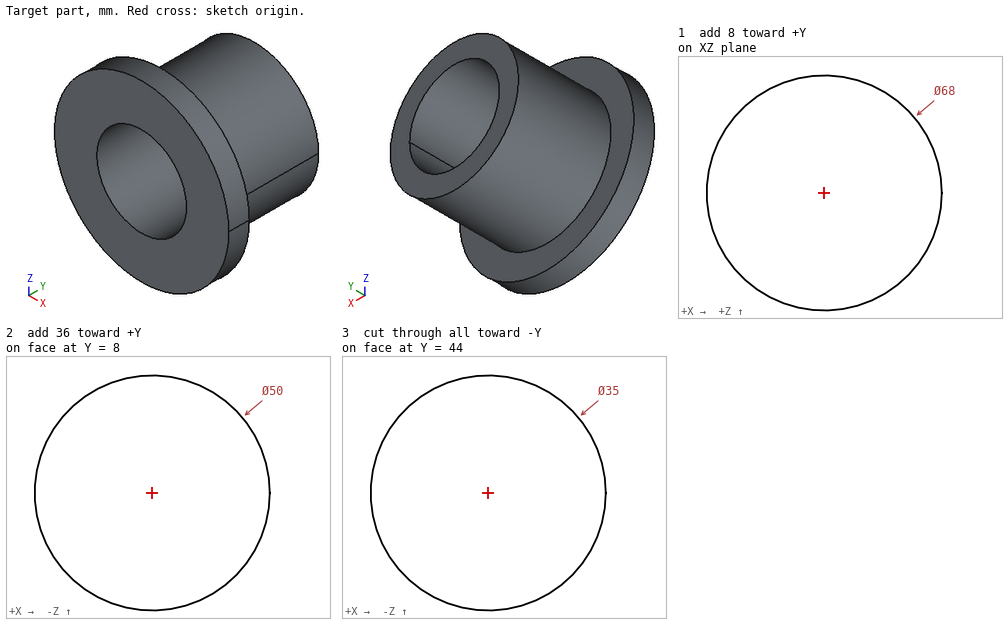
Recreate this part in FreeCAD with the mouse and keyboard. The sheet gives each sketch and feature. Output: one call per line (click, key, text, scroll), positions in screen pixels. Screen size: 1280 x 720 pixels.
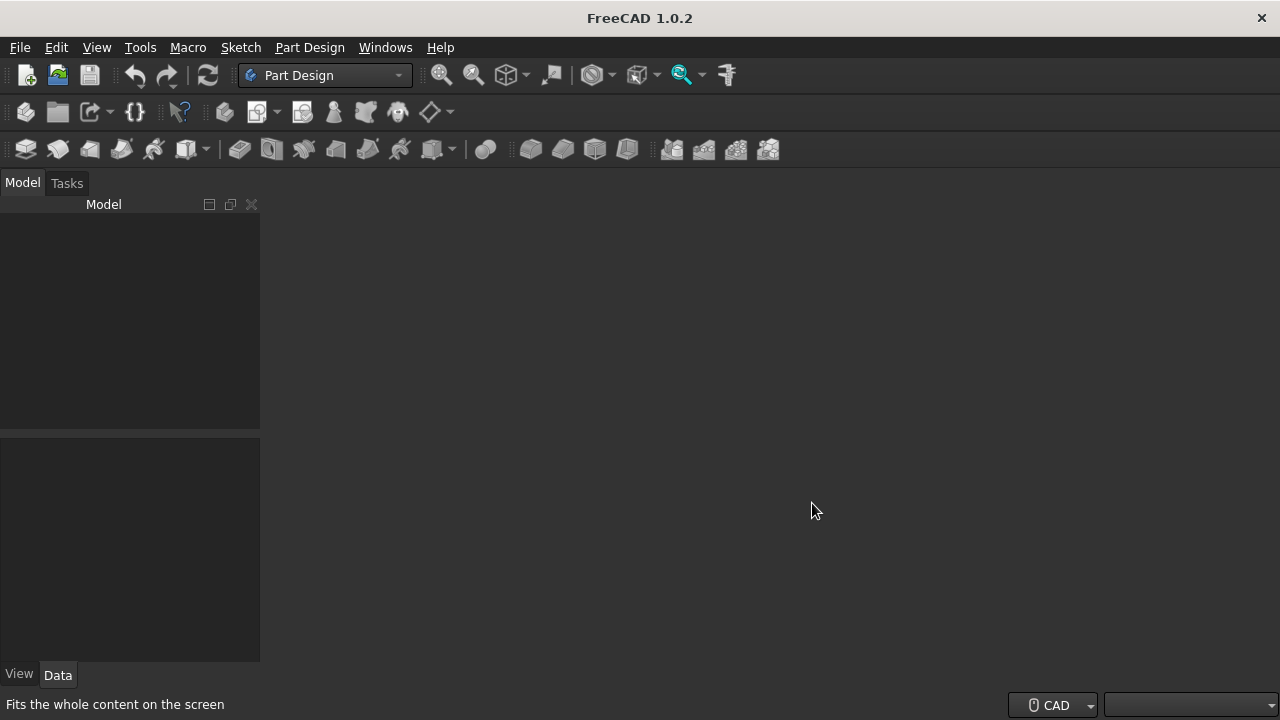
key(ctrl+n)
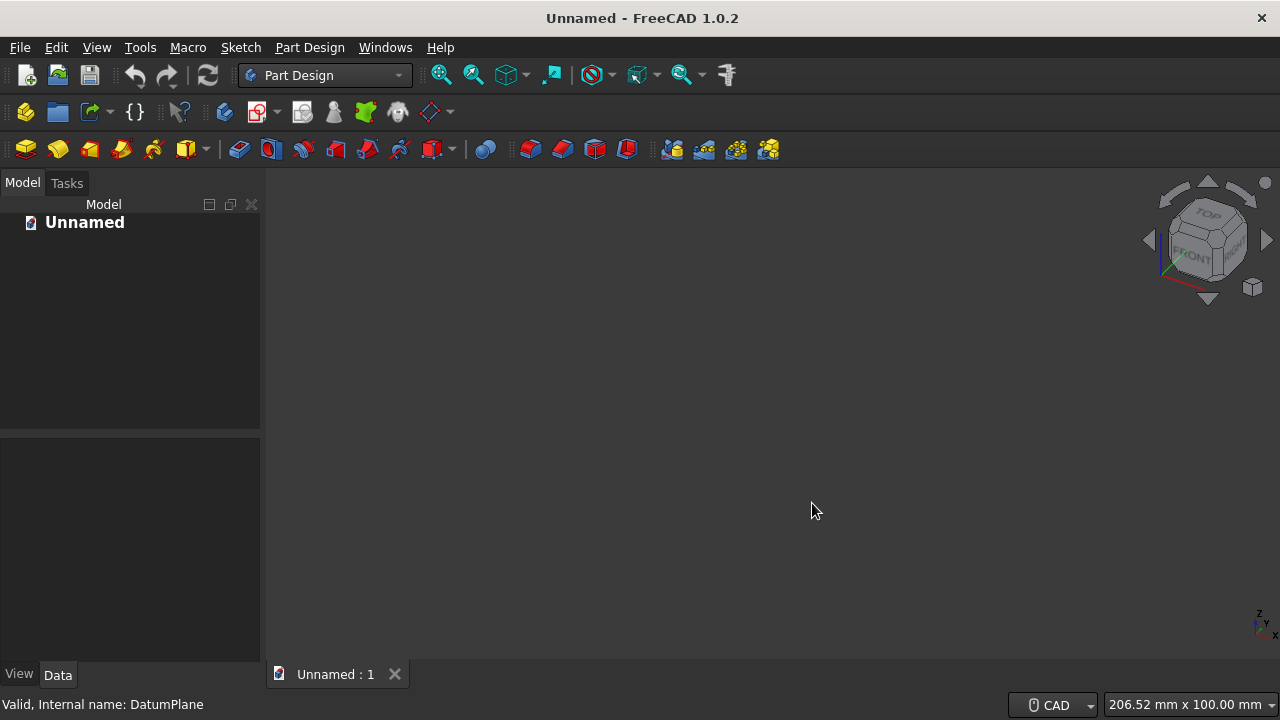
click(258, 112)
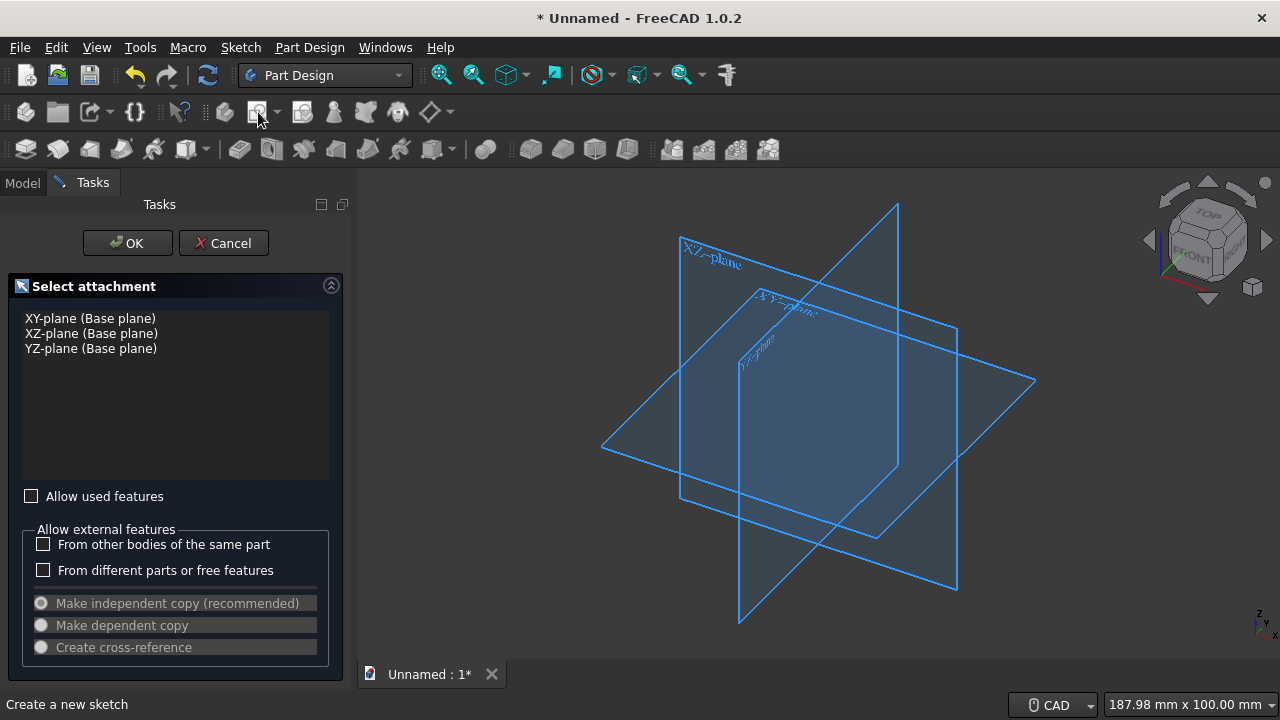
click(82, 334)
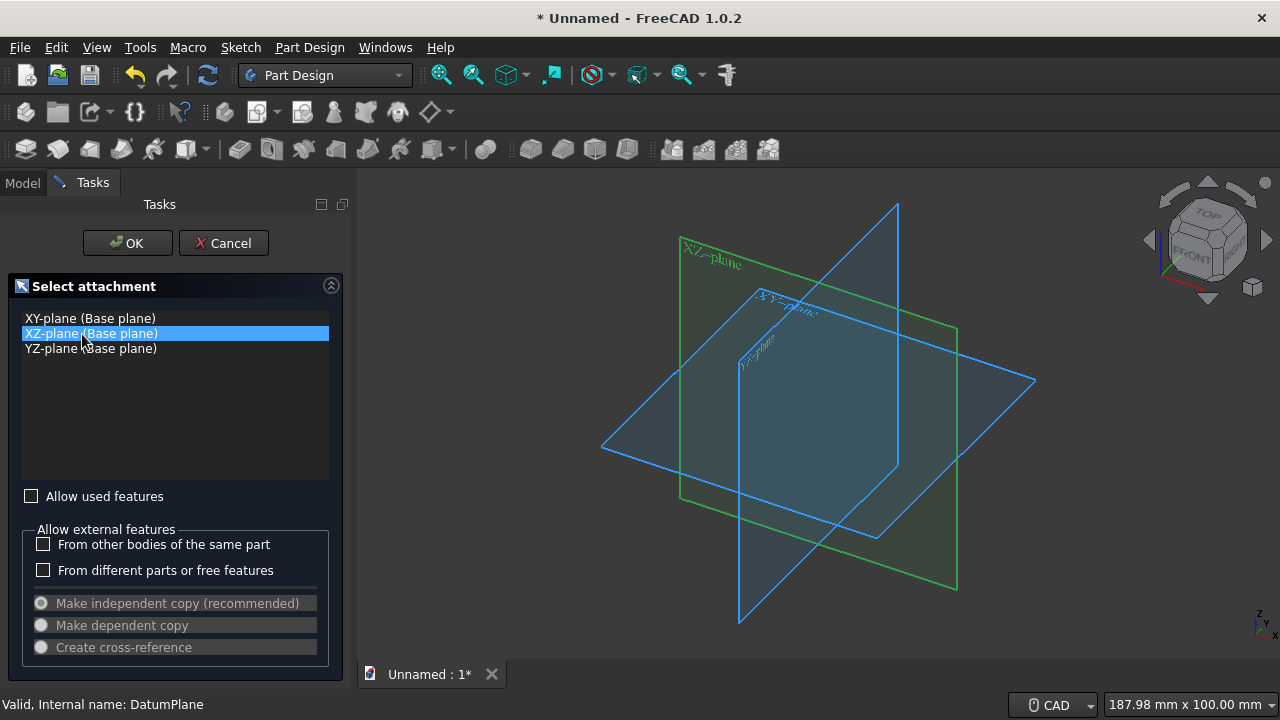
click(128, 243)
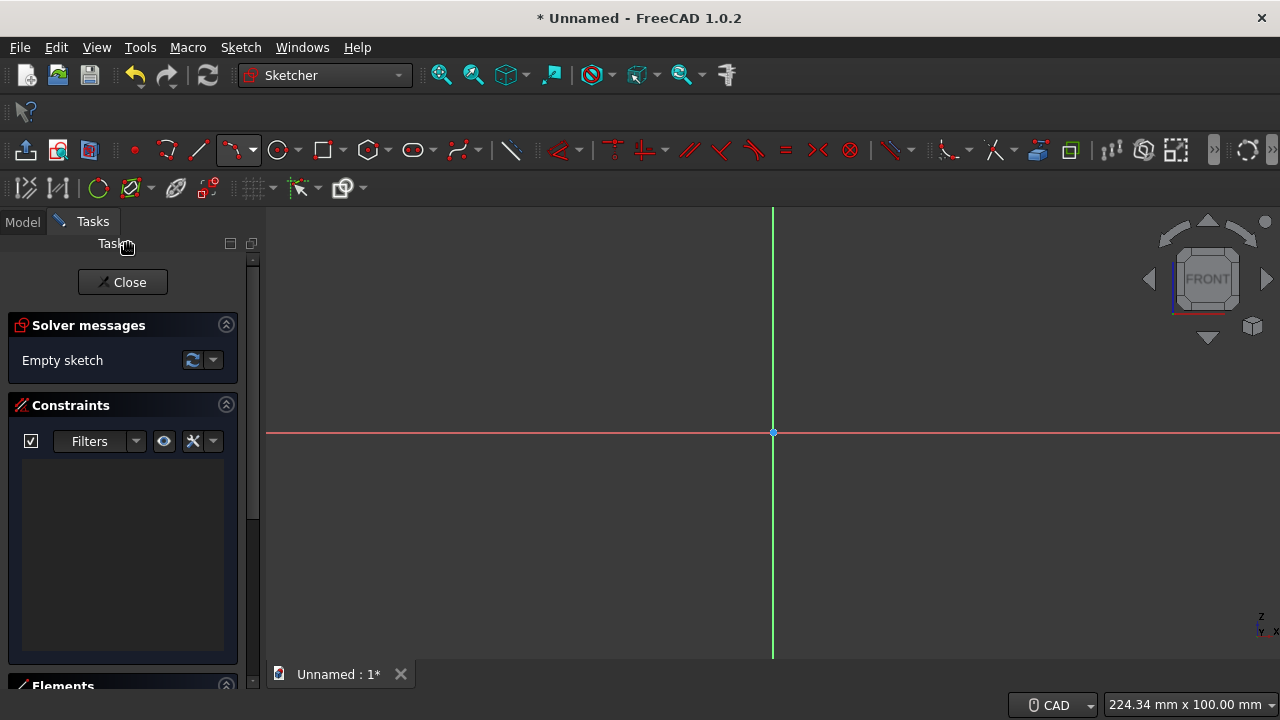
click(278, 150)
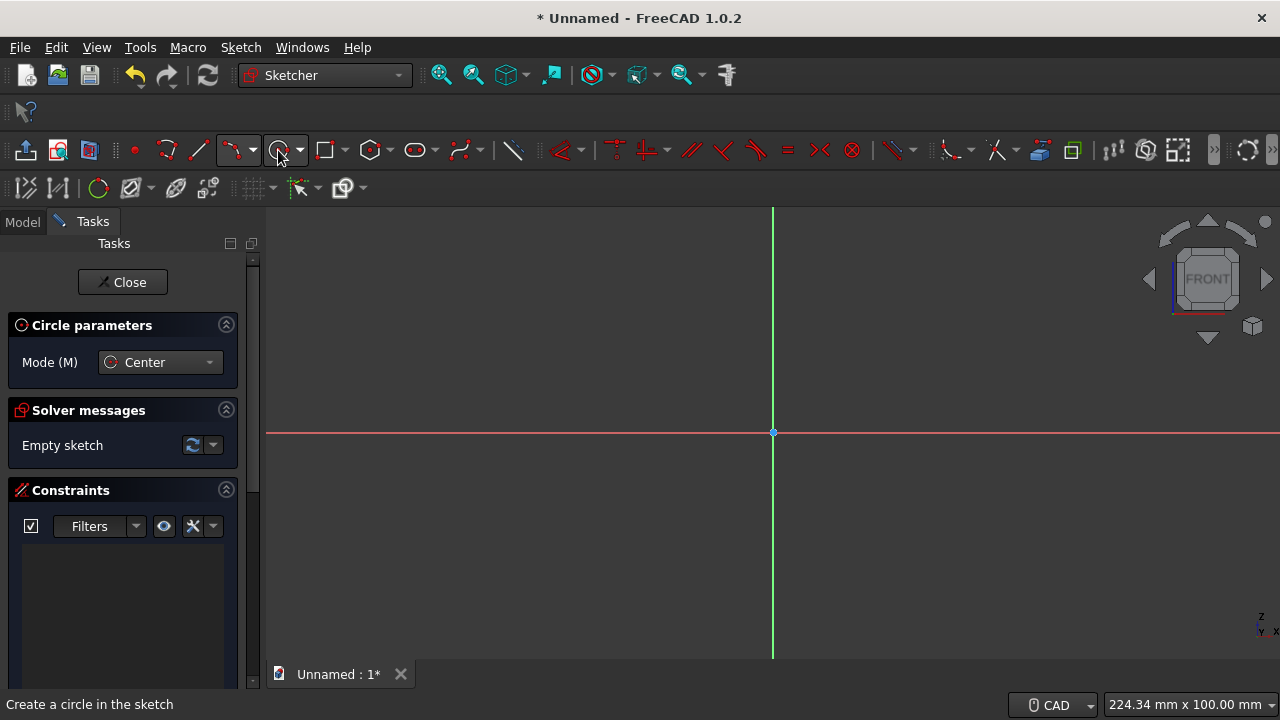
click(773, 433)
move(882, 324)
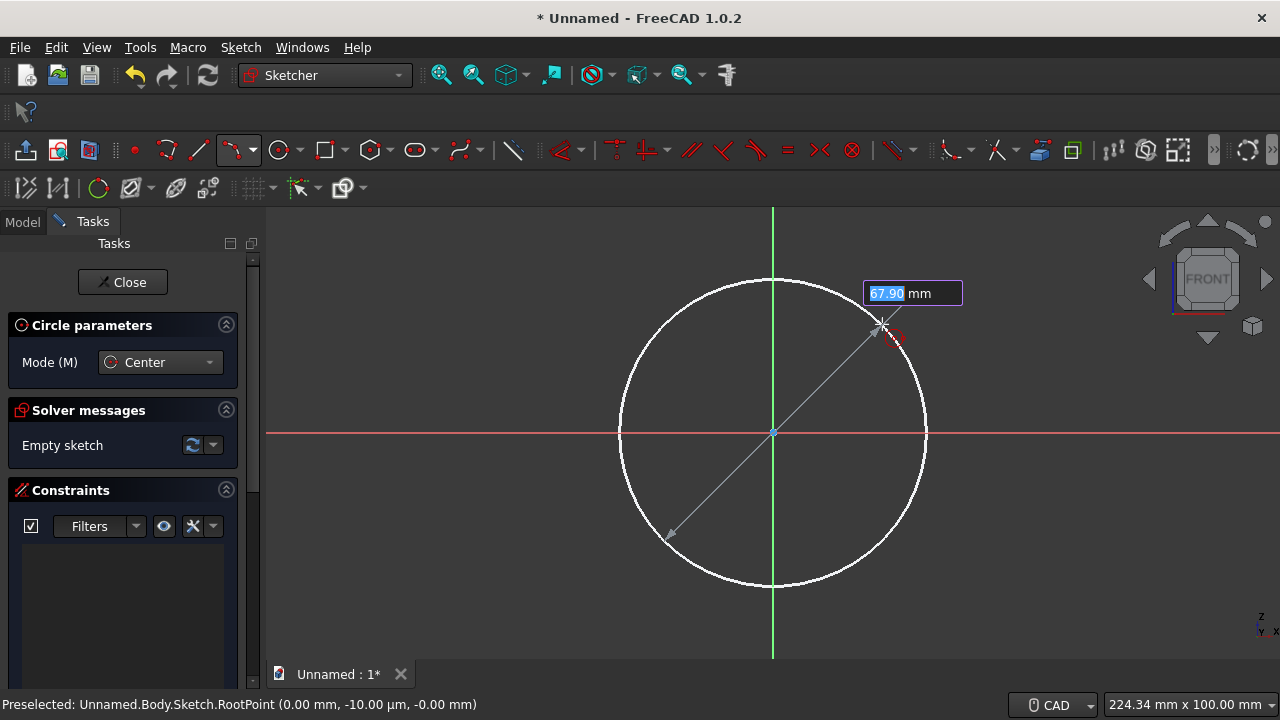
text(68)
key(Return)
key(Escape)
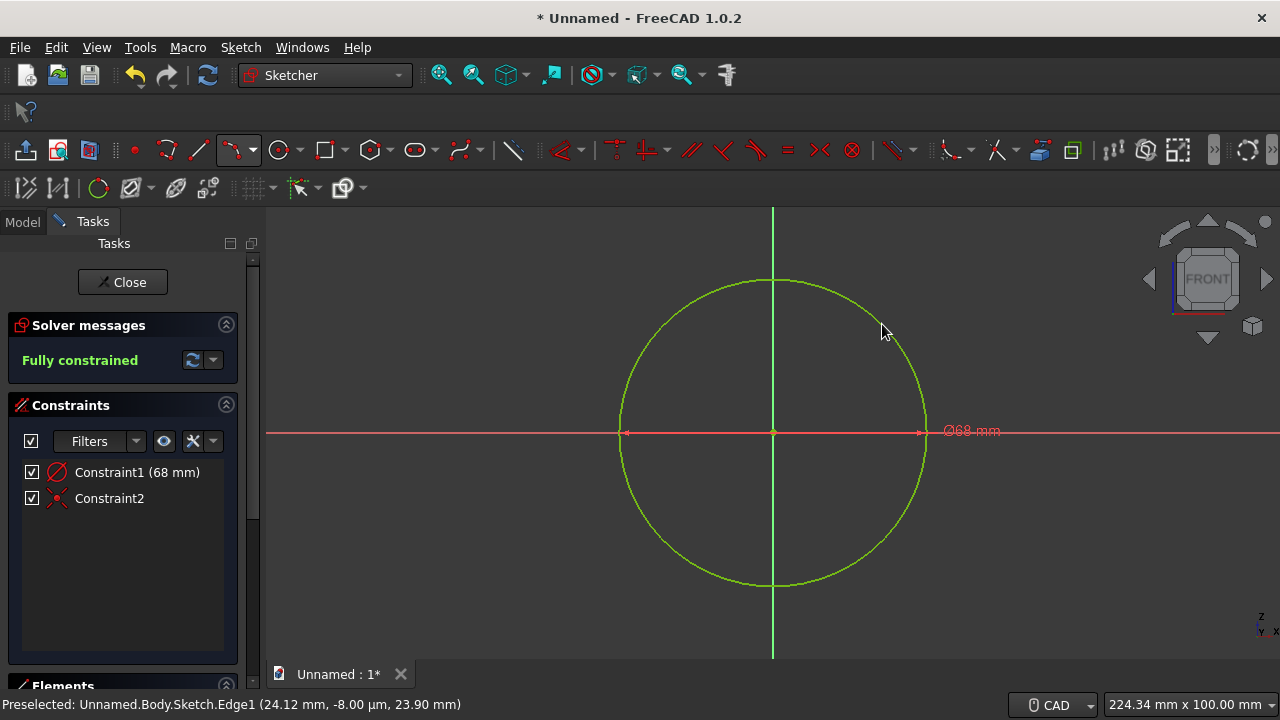
click(123, 282)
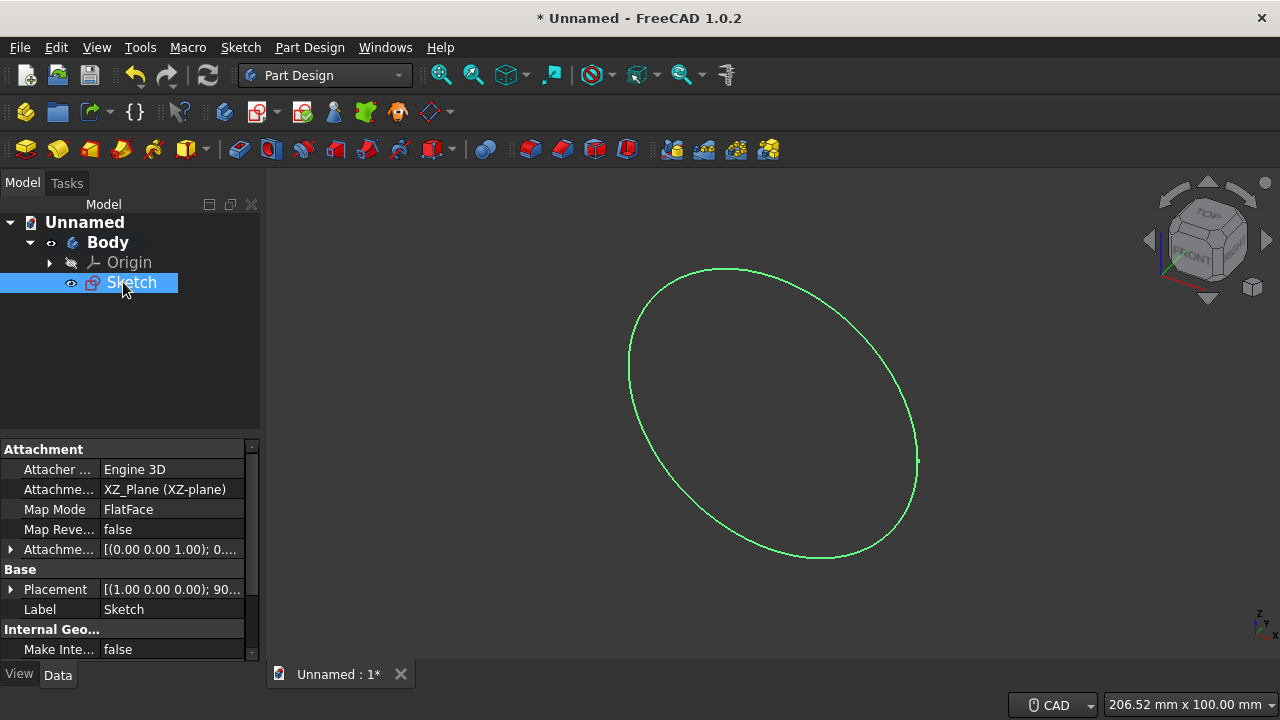
click(26, 150)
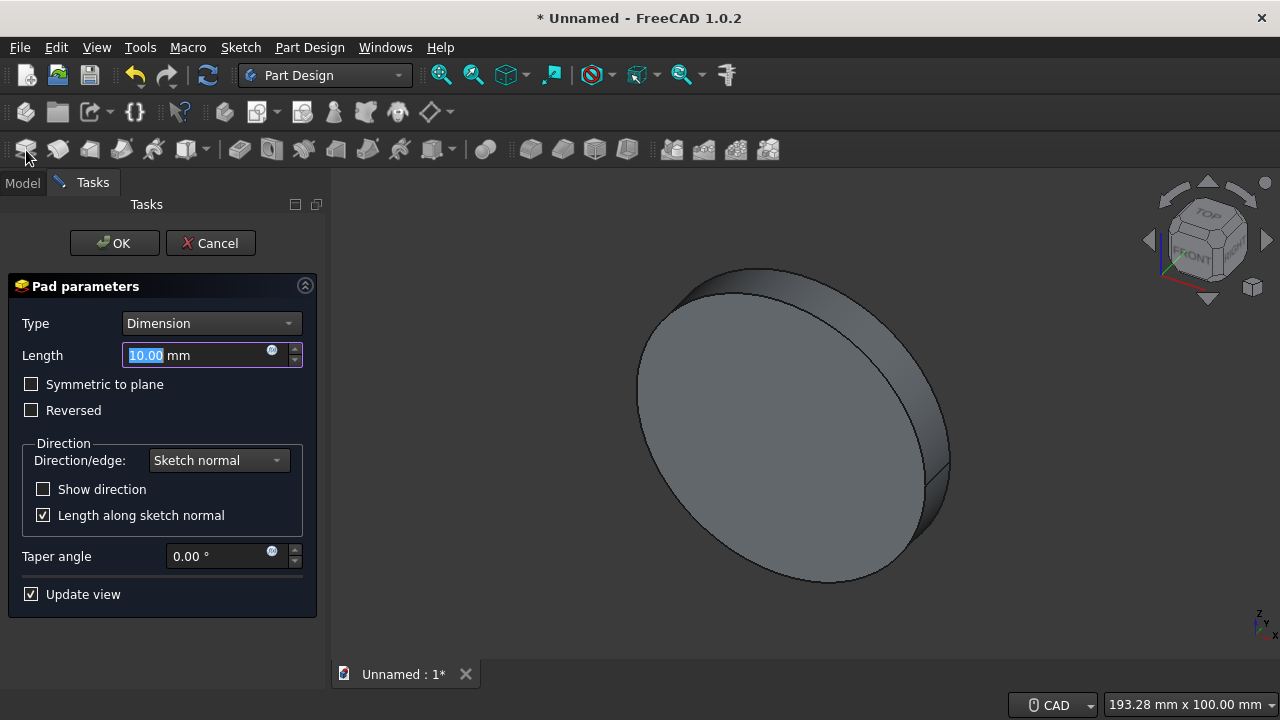
text(8)
key(Tab)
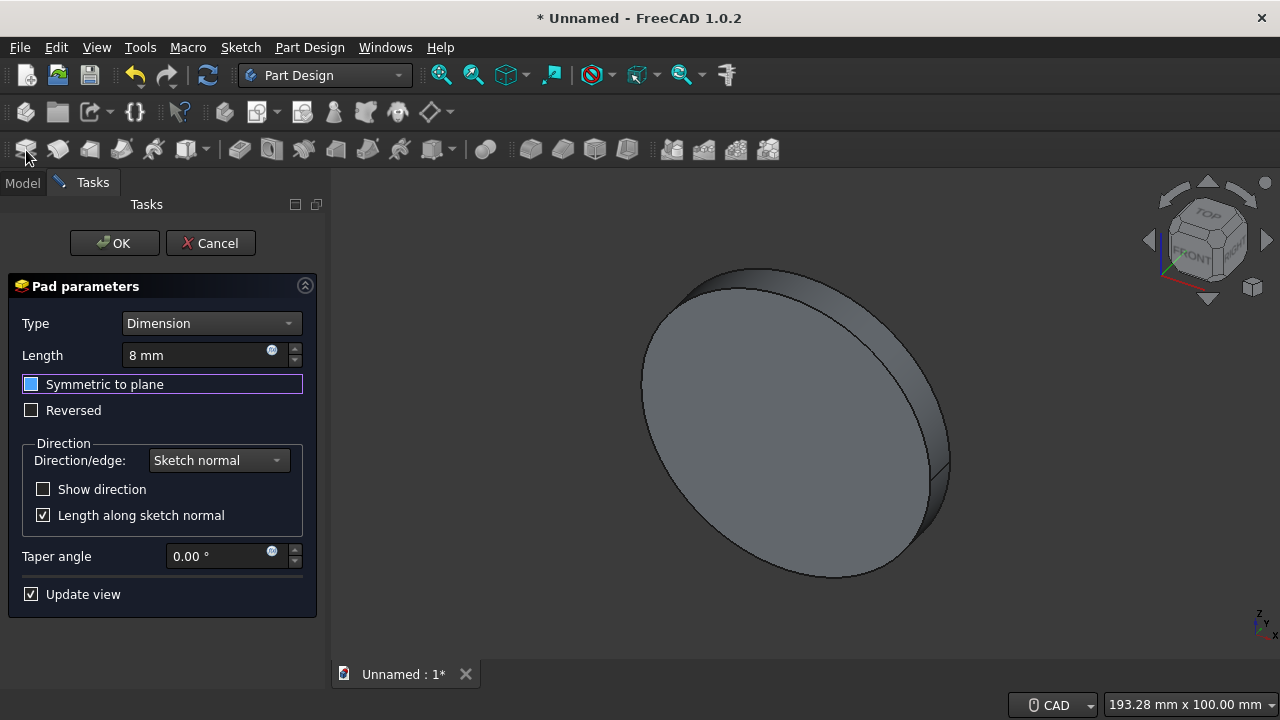
click(30, 410)